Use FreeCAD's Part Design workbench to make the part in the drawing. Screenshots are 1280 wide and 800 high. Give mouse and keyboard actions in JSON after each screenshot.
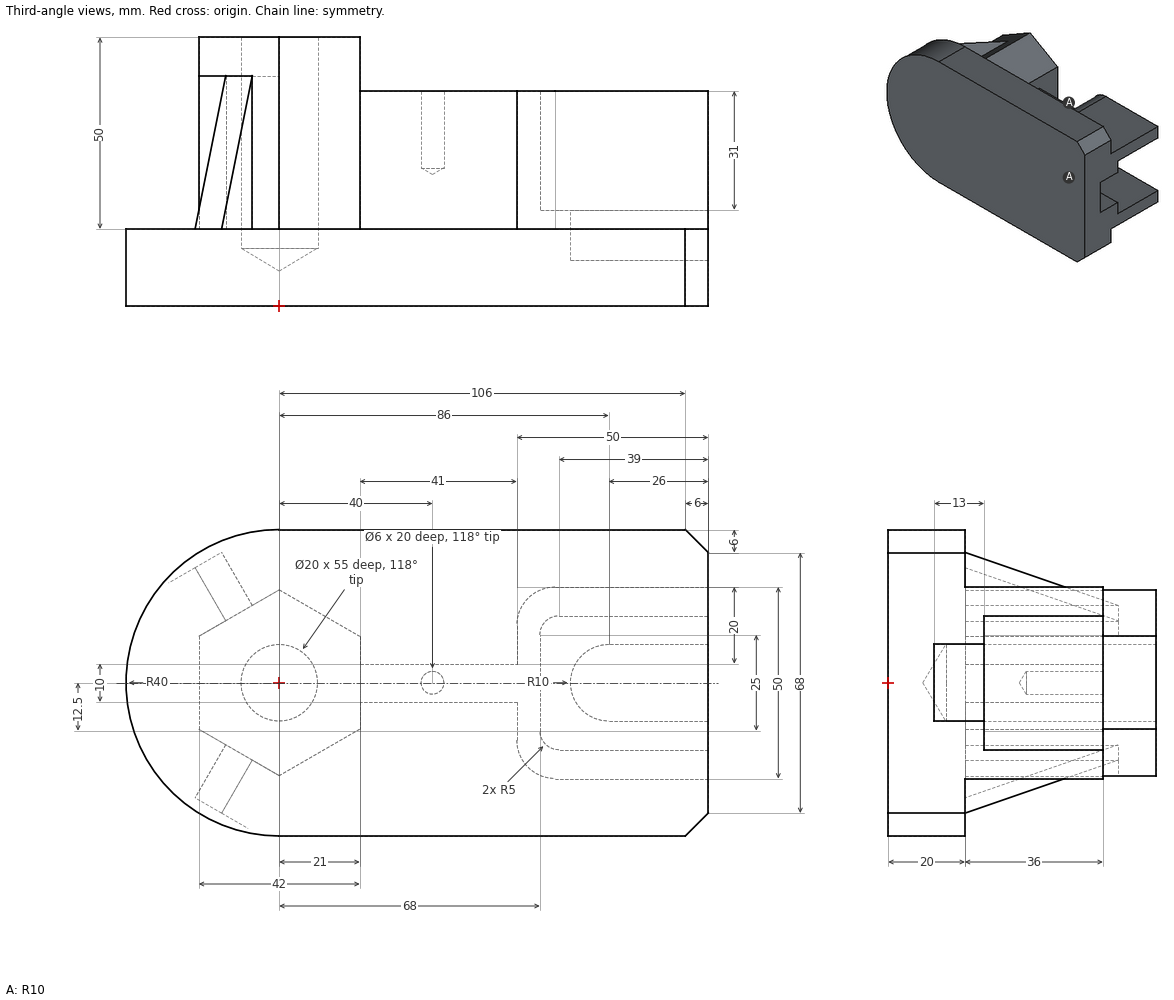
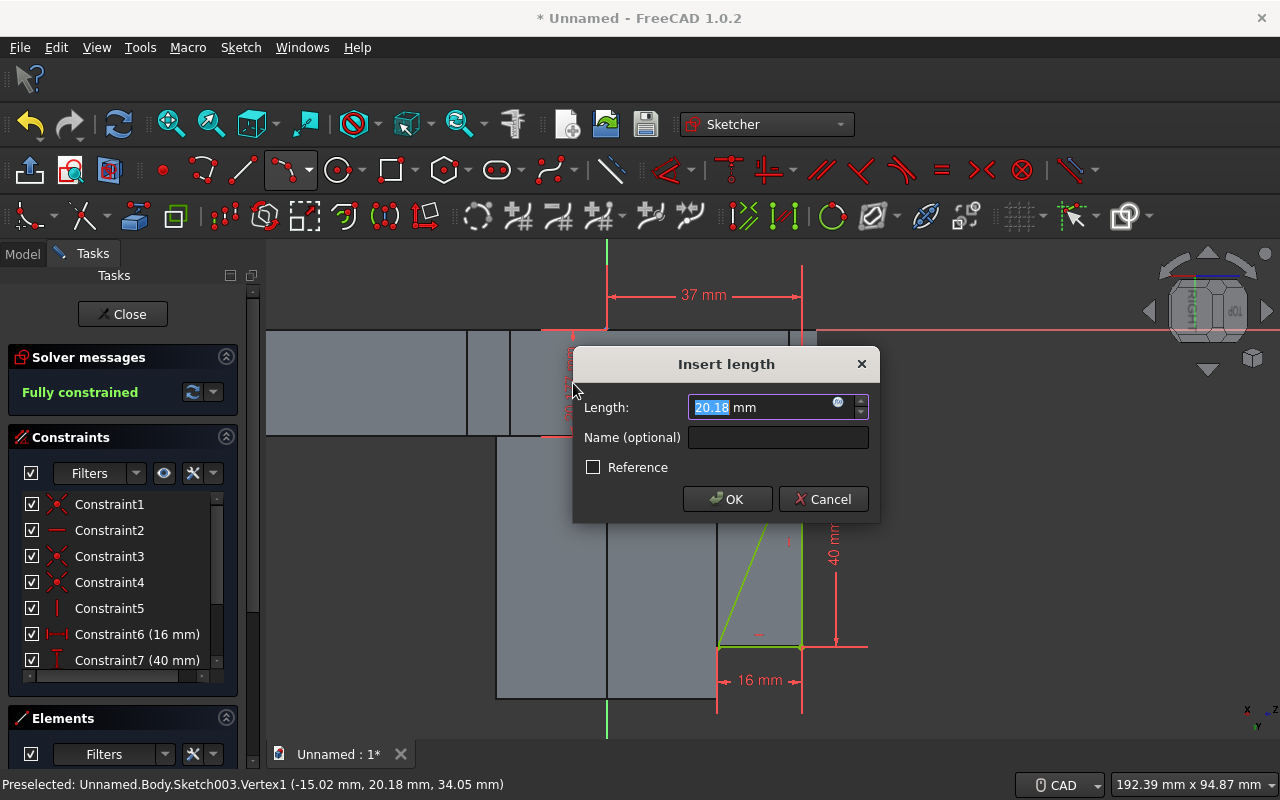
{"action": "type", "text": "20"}
{"action": "key", "text": "Return"}
{"action": "key", "text": "Escape"}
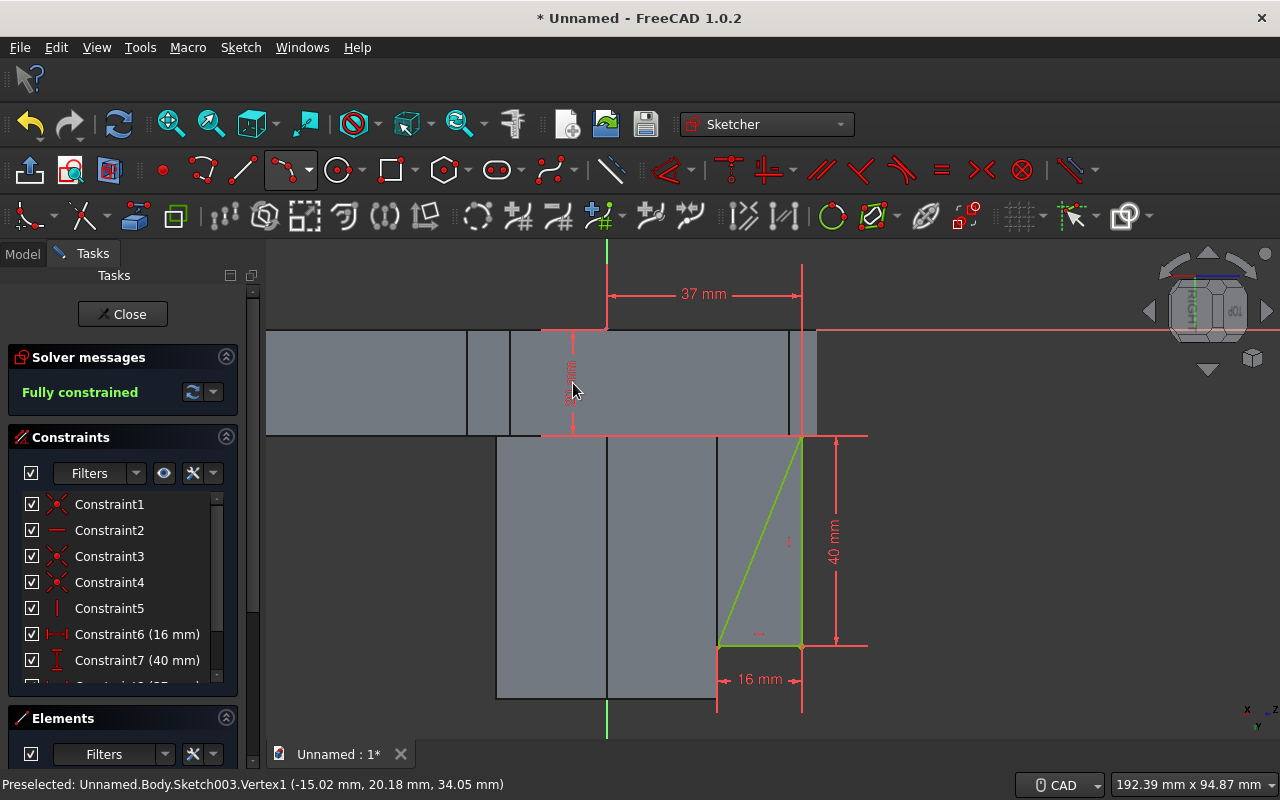
{"action": "left_click", "coordinate": [123, 314]}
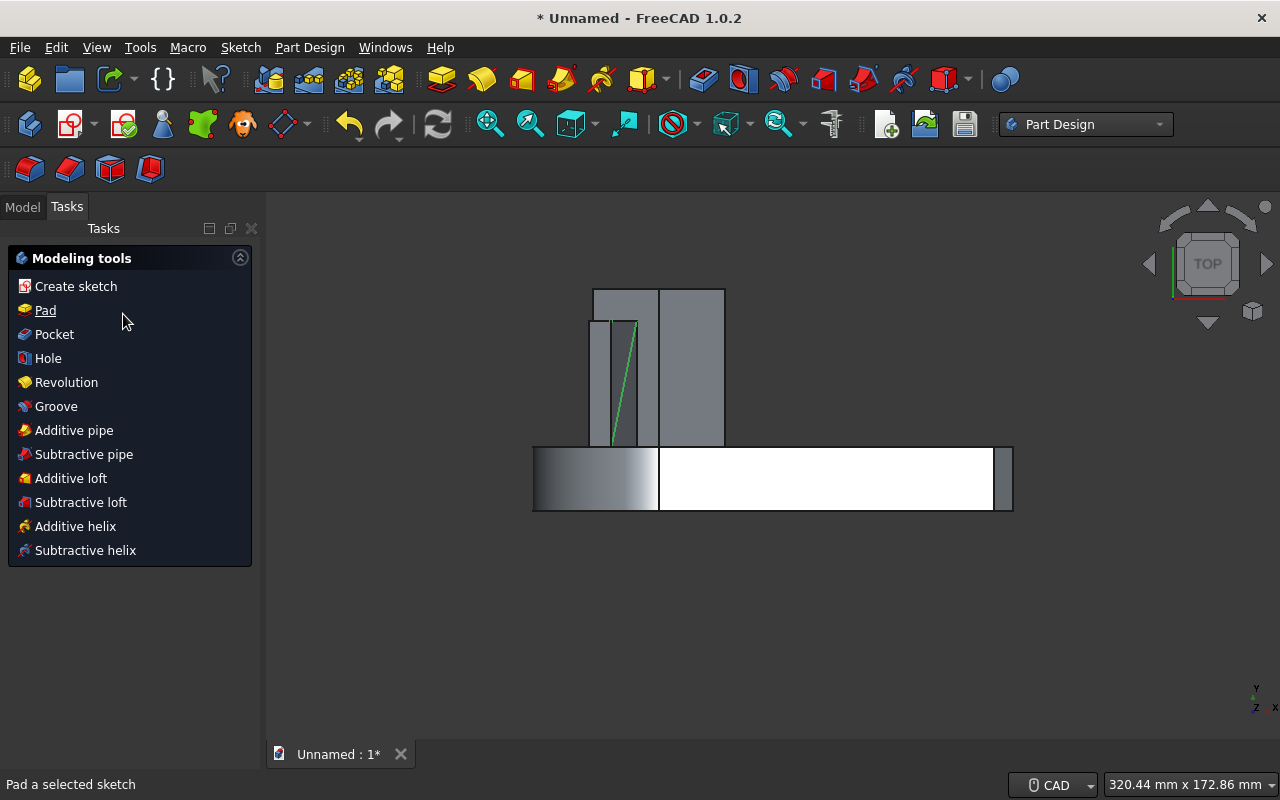
{"action": "left_click", "coordinate": [704, 80]}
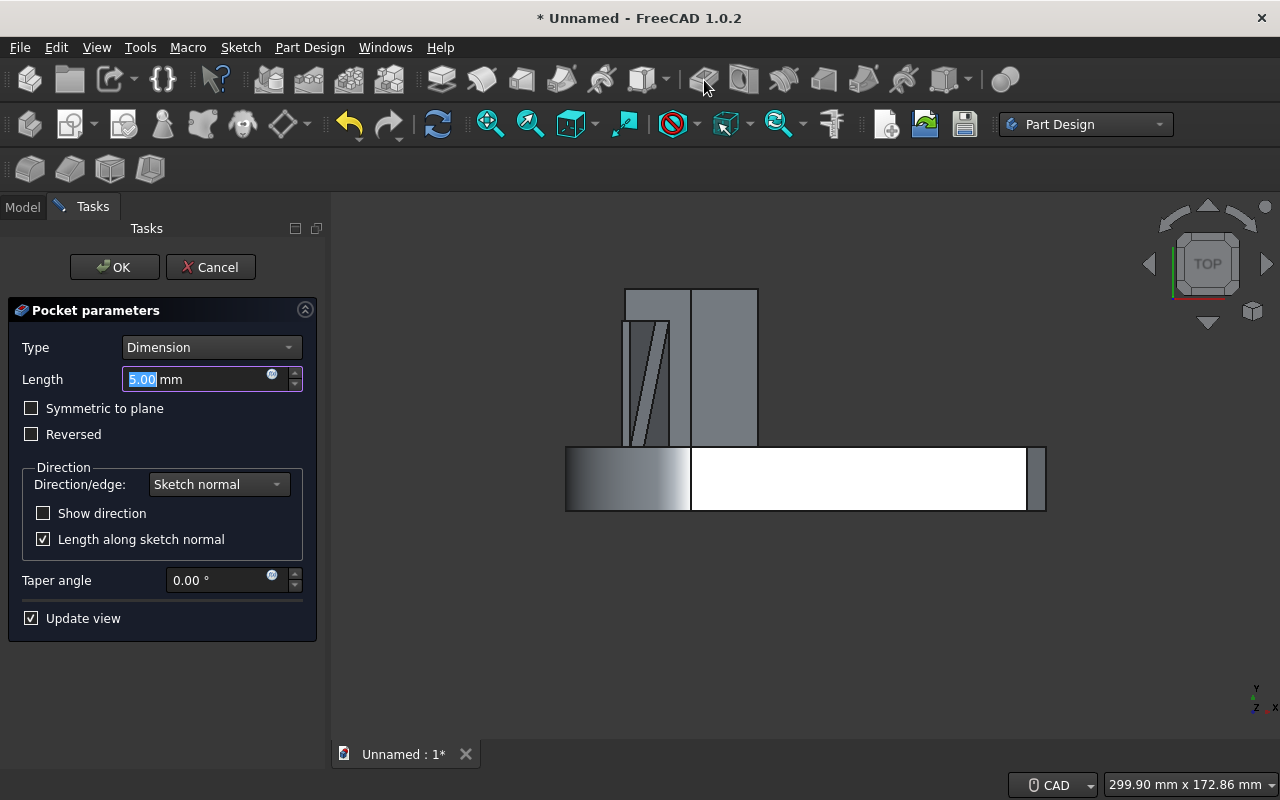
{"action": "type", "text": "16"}
{"action": "key", "text": "Tab"}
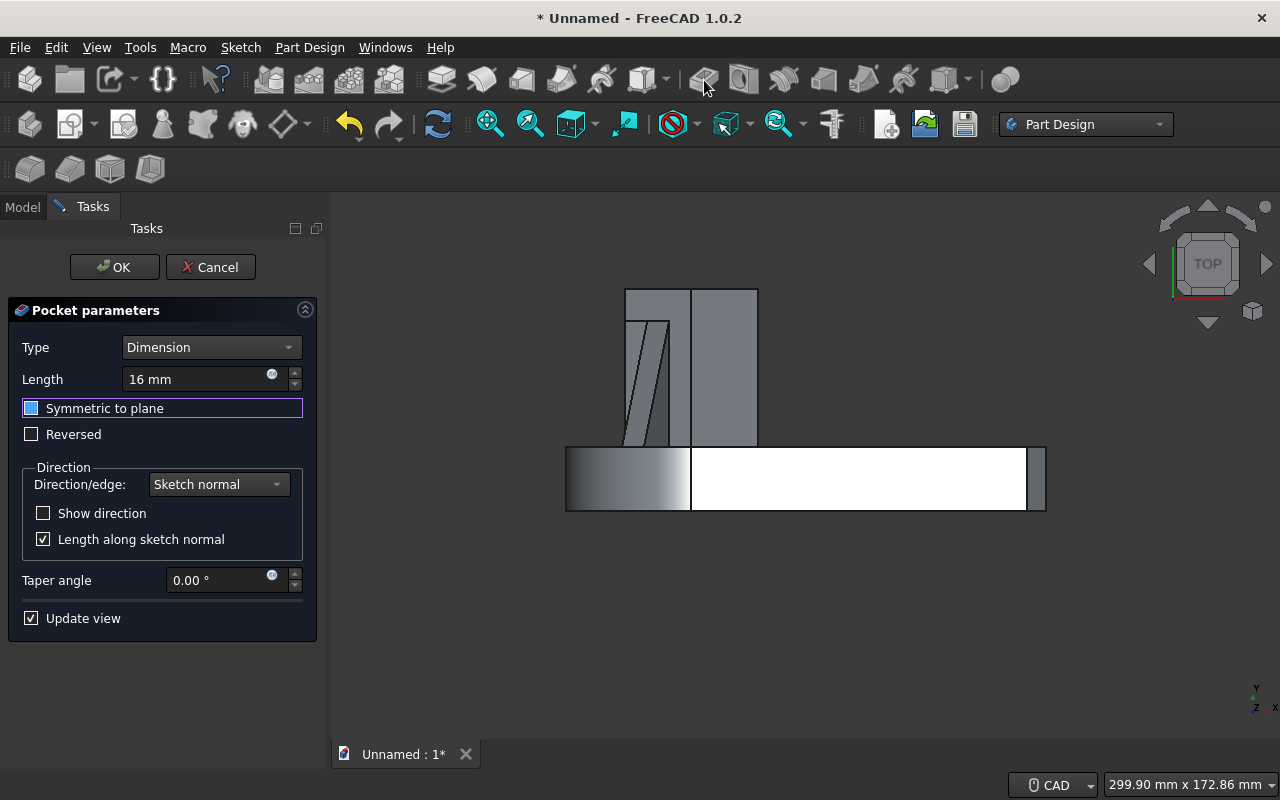
{"action": "left_click", "coordinate": [115, 267]}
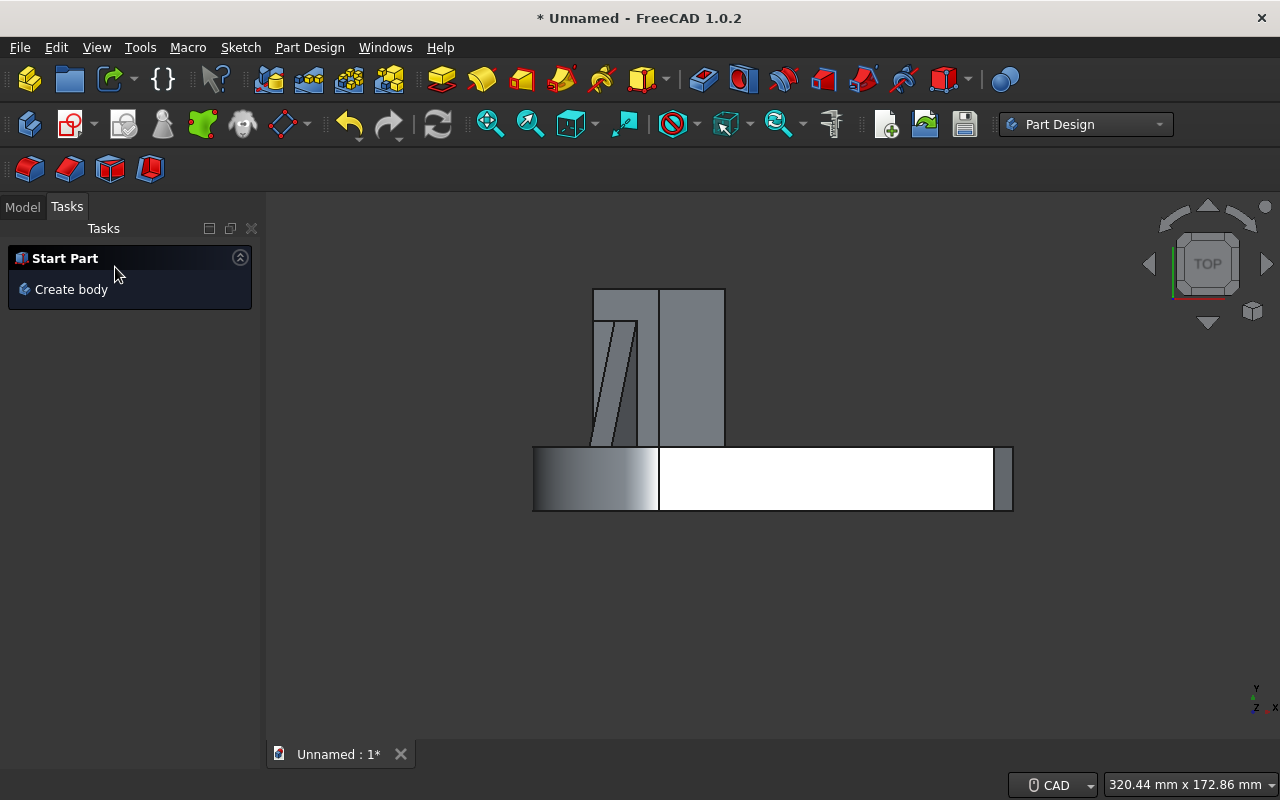
{"action": "key", "text": "5"}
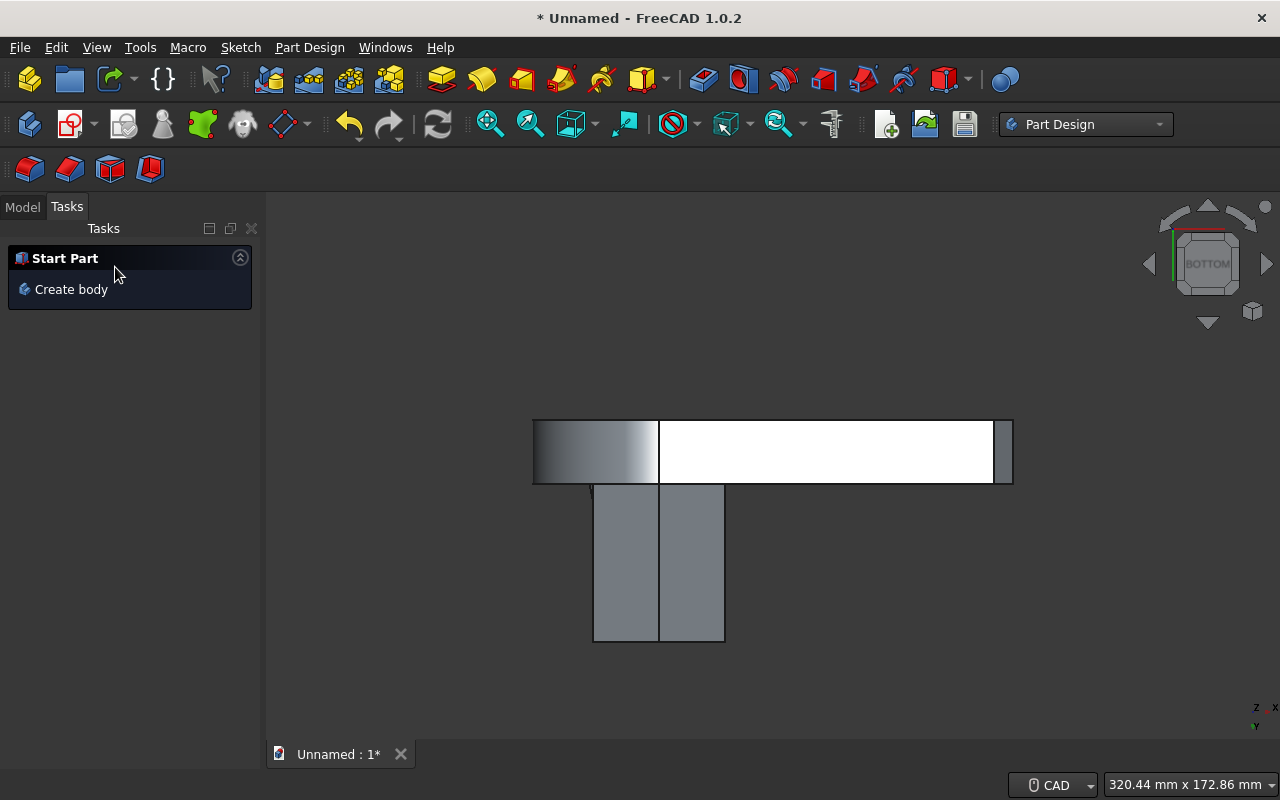
{"action": "left_click", "coordinate": [626, 584]}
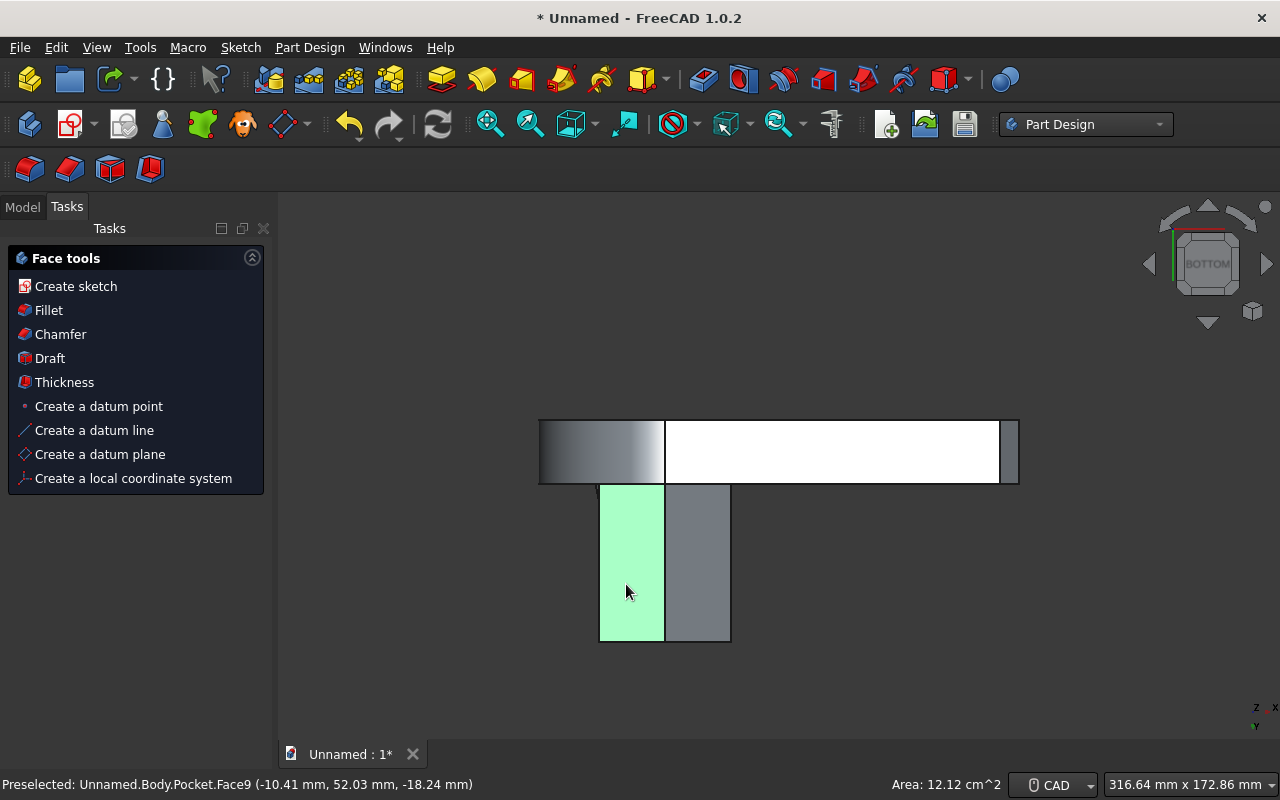
{"action": "left_click", "coordinate": [70, 124]}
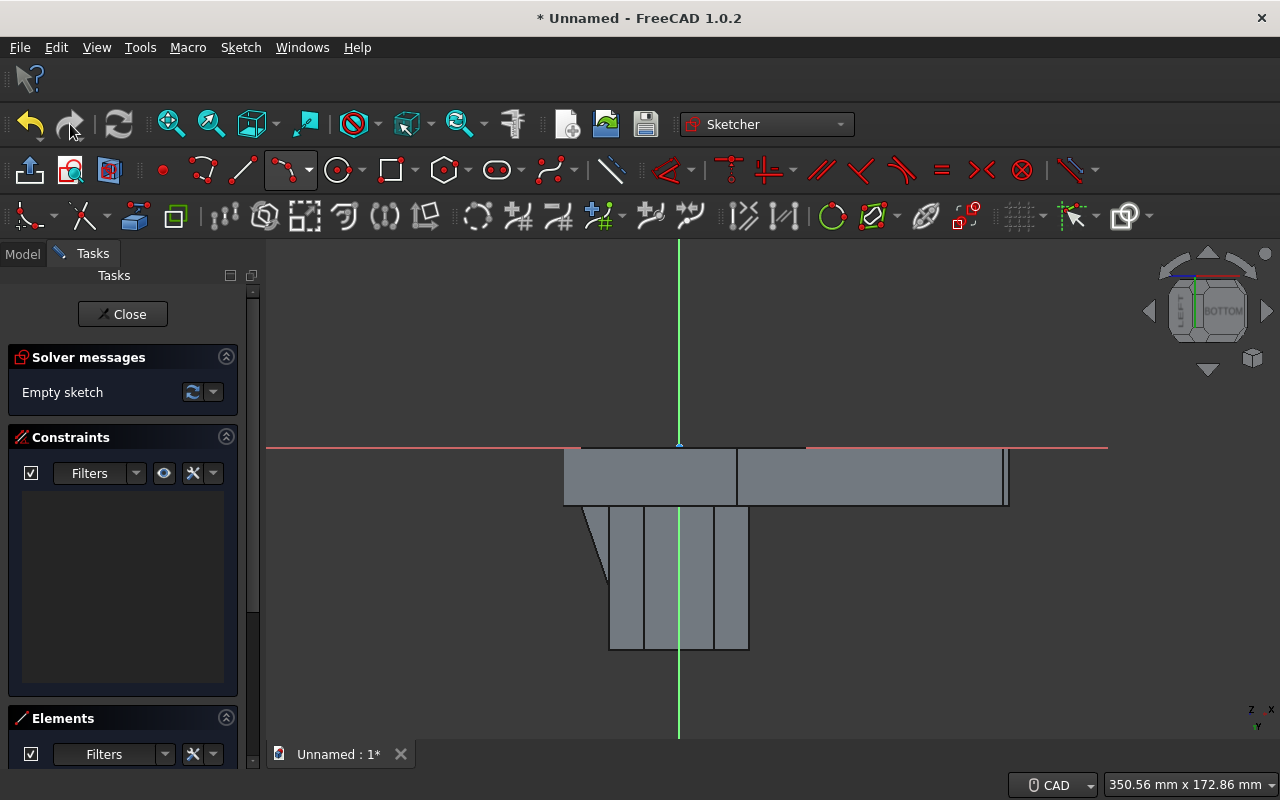
{"action": "left_click", "coordinate": [110, 170]}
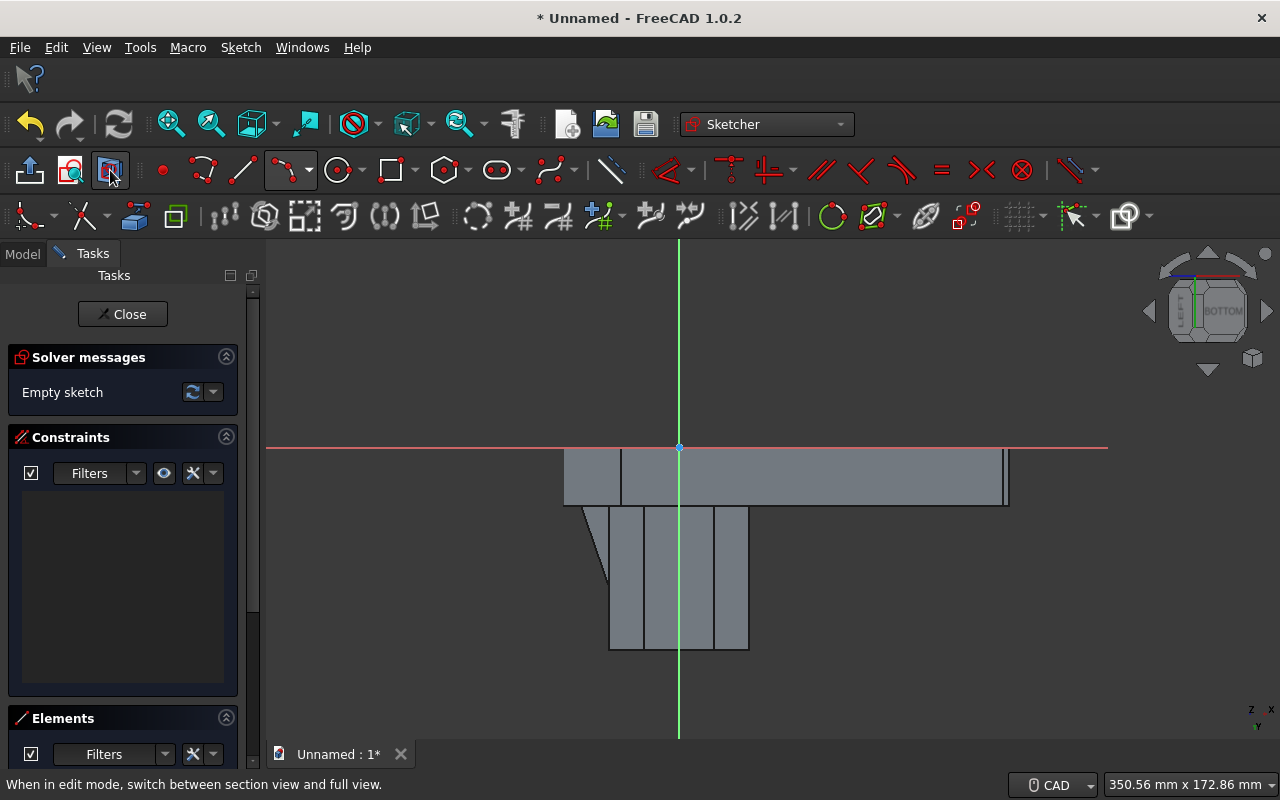
{"action": "scroll", "coordinate": [649, 590], "scroll_direction": "up", "scroll_amount": 3}